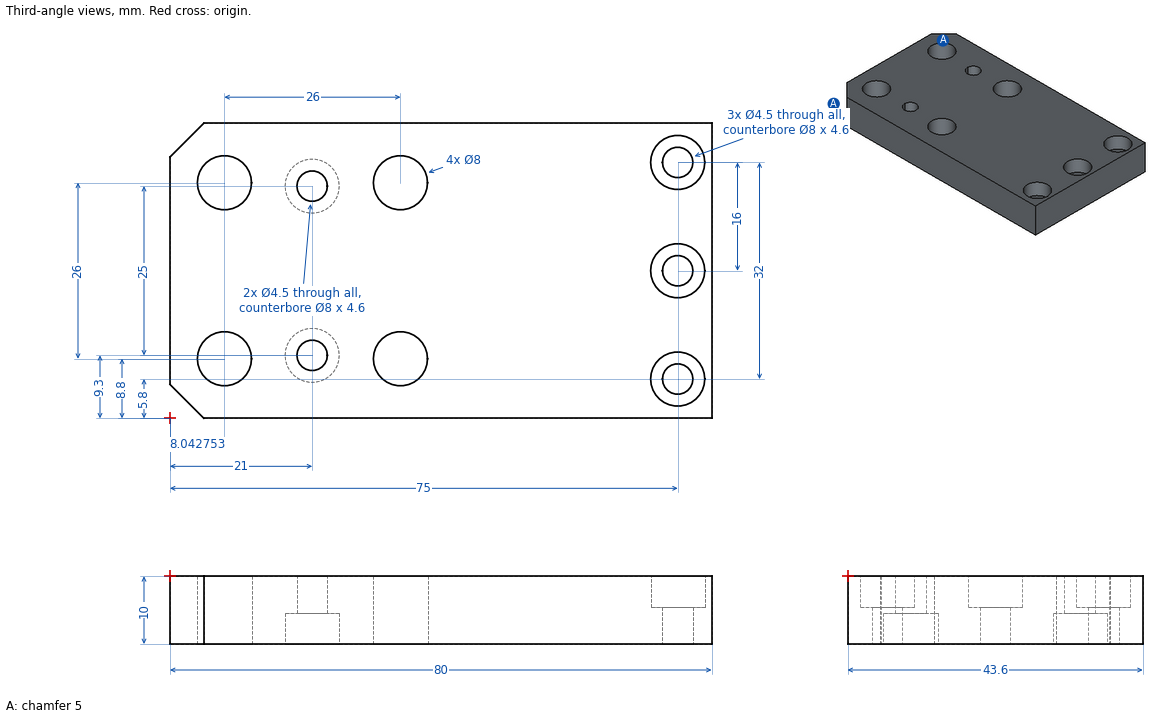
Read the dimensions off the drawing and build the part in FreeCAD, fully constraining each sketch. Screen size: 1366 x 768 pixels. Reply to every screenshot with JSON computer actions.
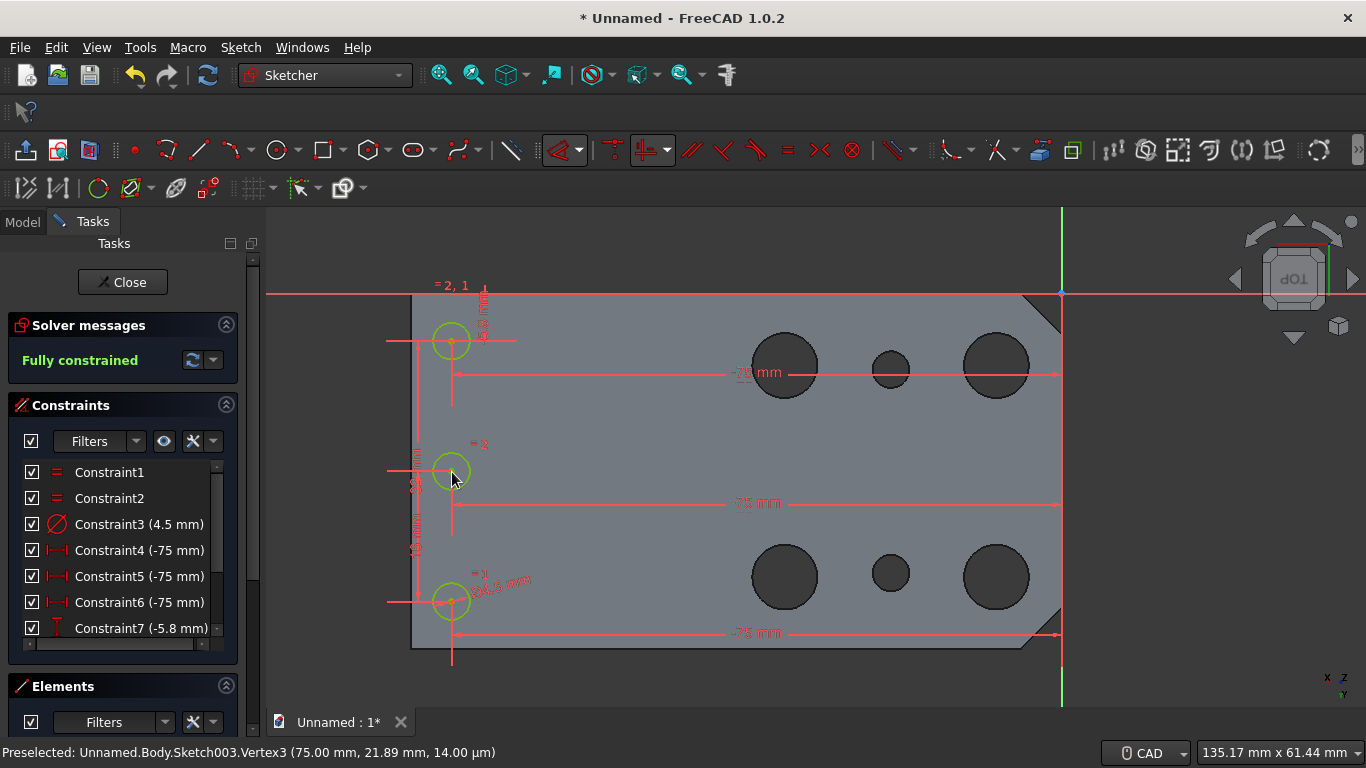
{"action": "left_click", "coordinate": [123, 282]}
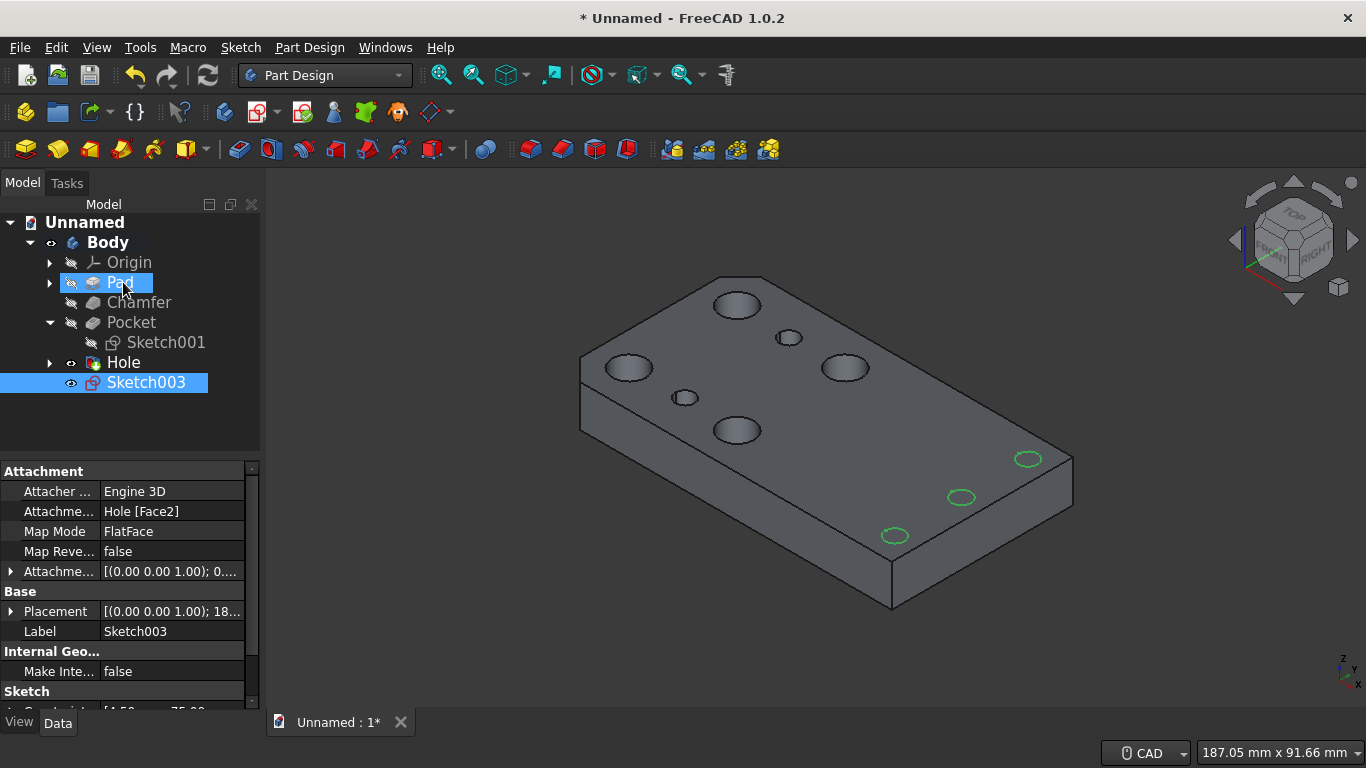
{"action": "left_click", "coordinate": [272, 150]}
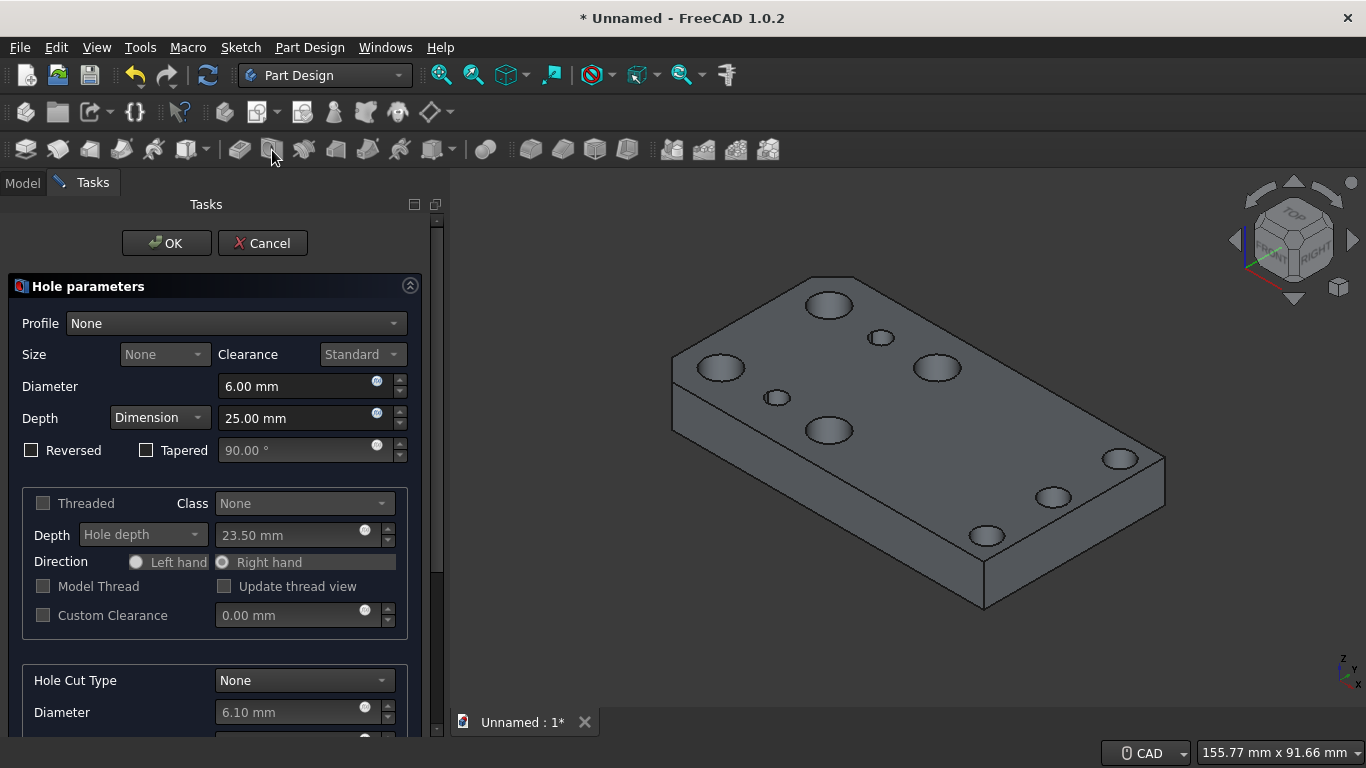
{"action": "triple_click", "coordinate": [305, 386]}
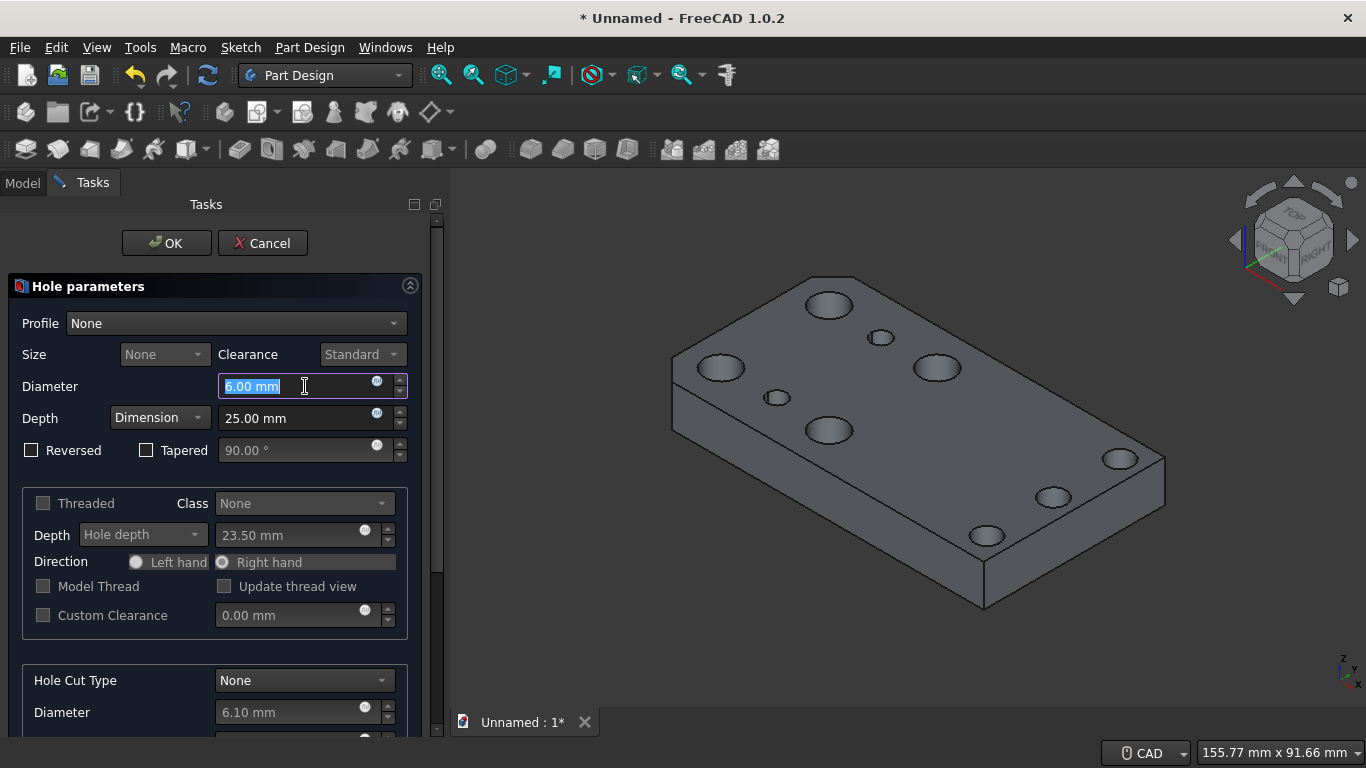
{"action": "type", "text": "4.5"}
{"action": "key", "text": "Tab"}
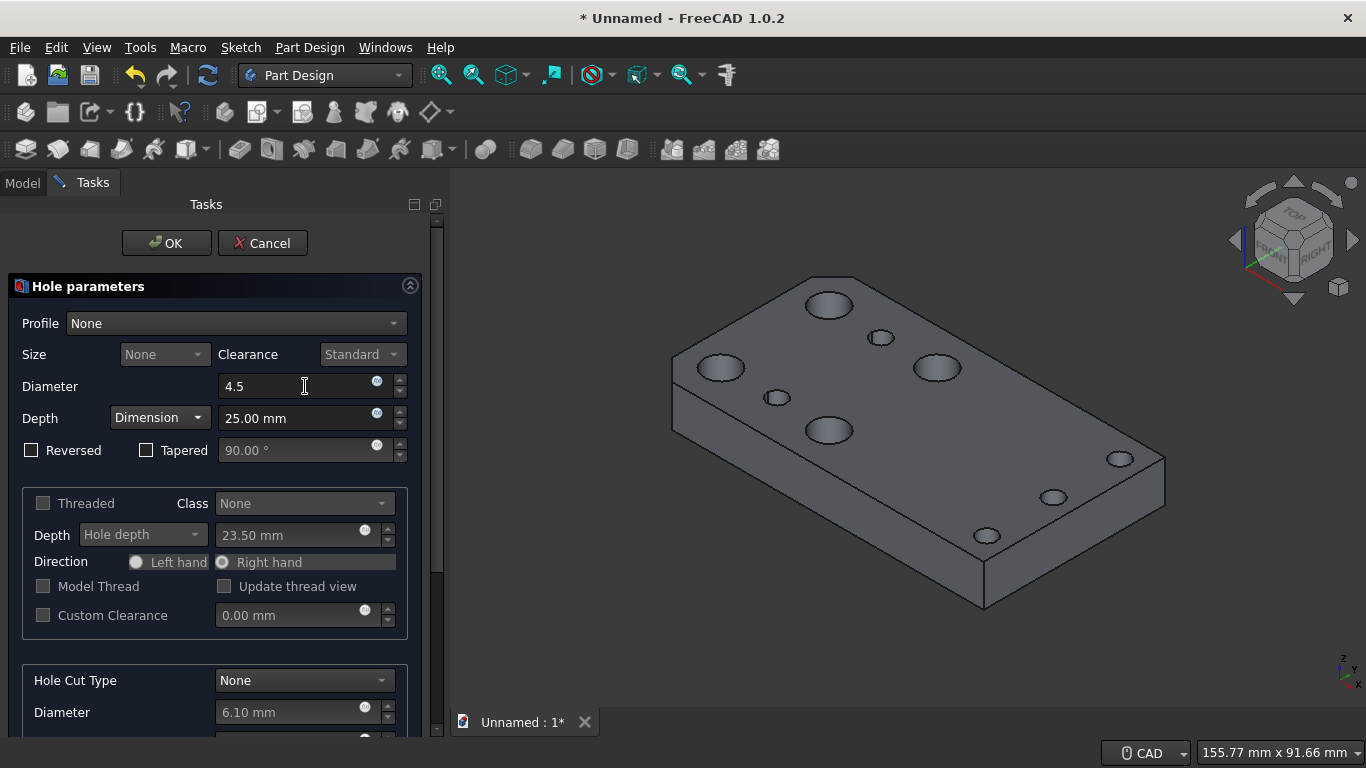
{"action": "left_click", "coordinate": [161, 418]}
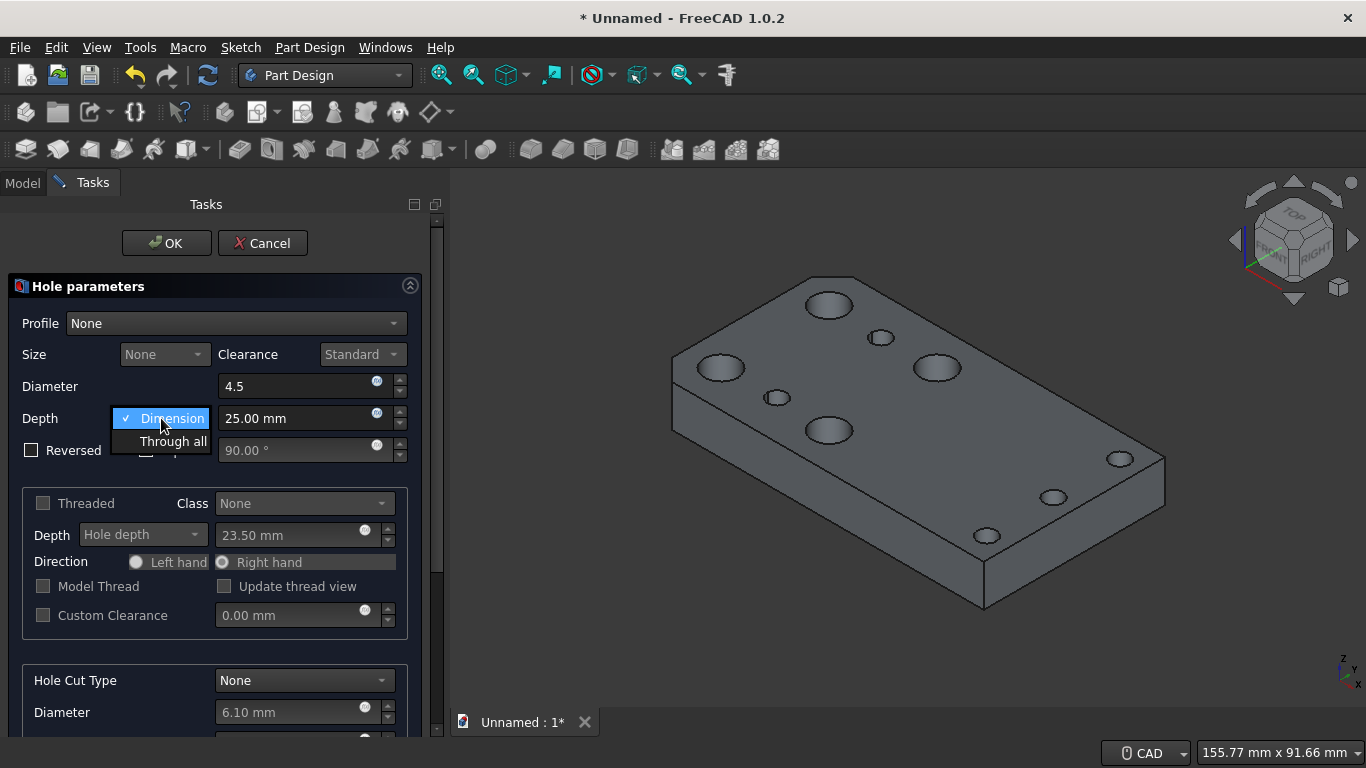
{"action": "left_click", "coordinate": [160, 442]}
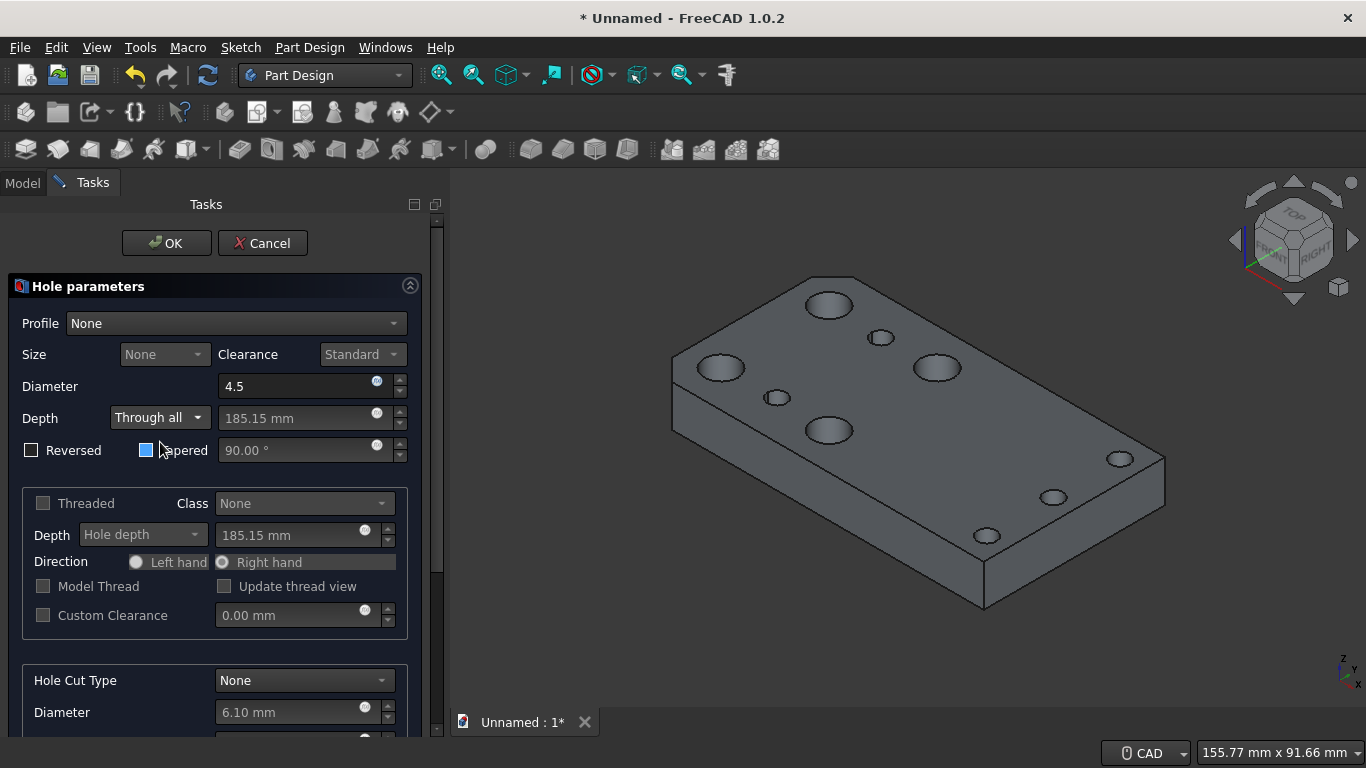
{"action": "left_click", "coordinate": [306, 680]}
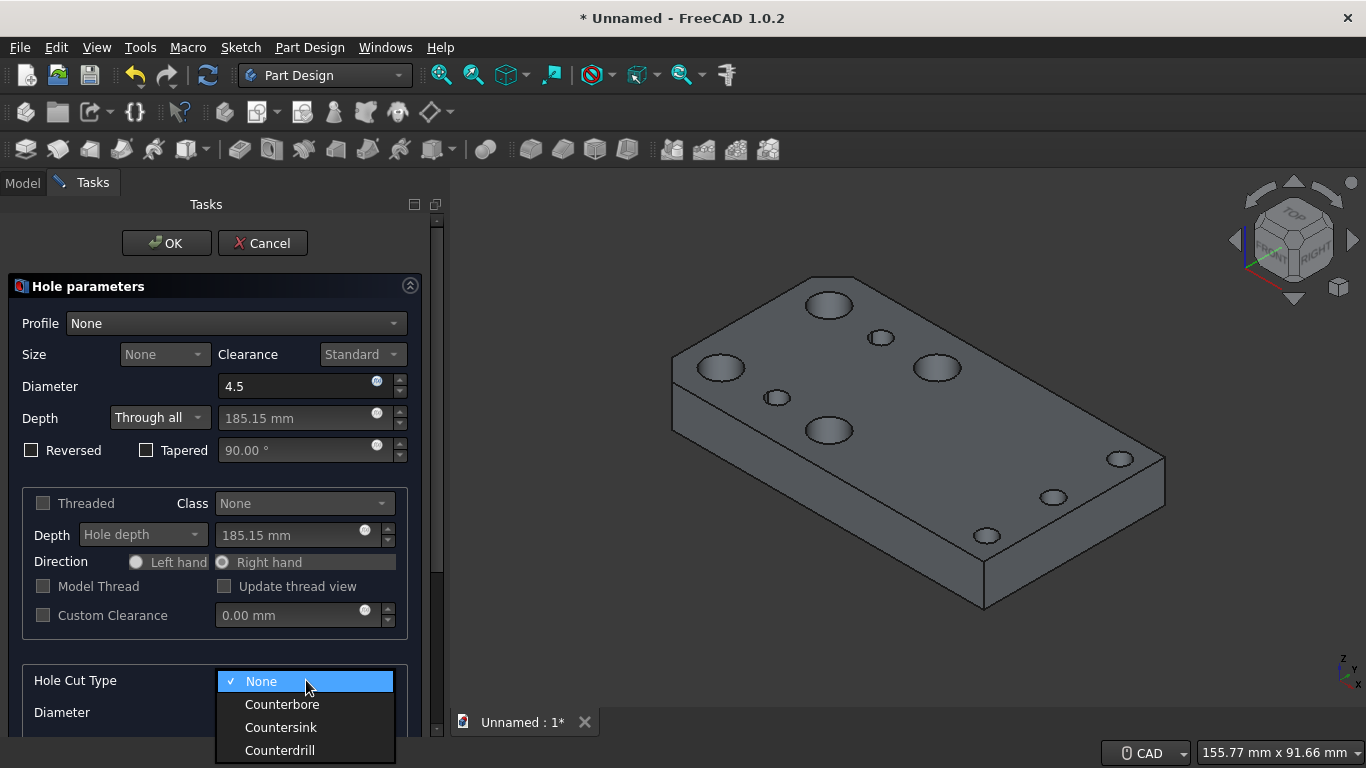
{"action": "left_click", "coordinate": [304, 704]}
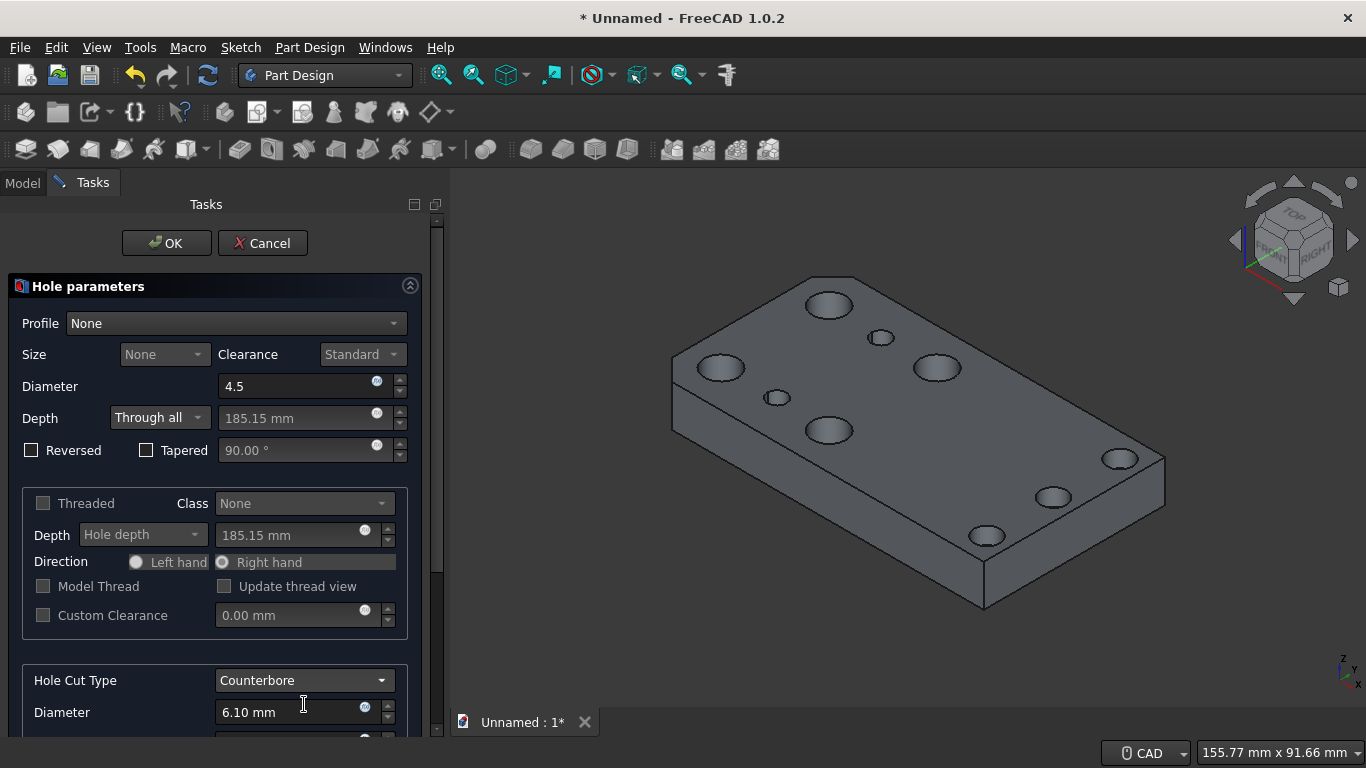
{"action": "triple_click", "coordinate": [298, 712]}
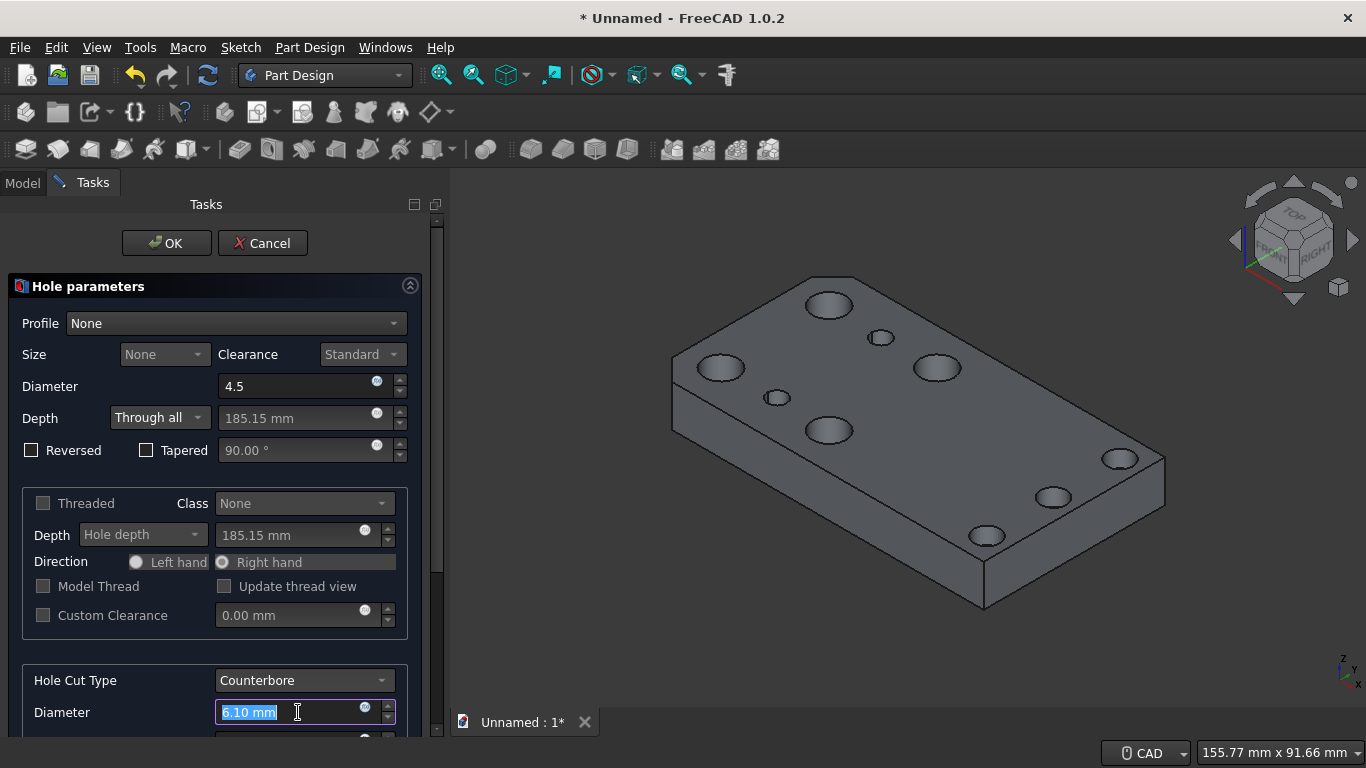
{"action": "type", "text": "8"}
{"action": "key", "text": "Tab"}